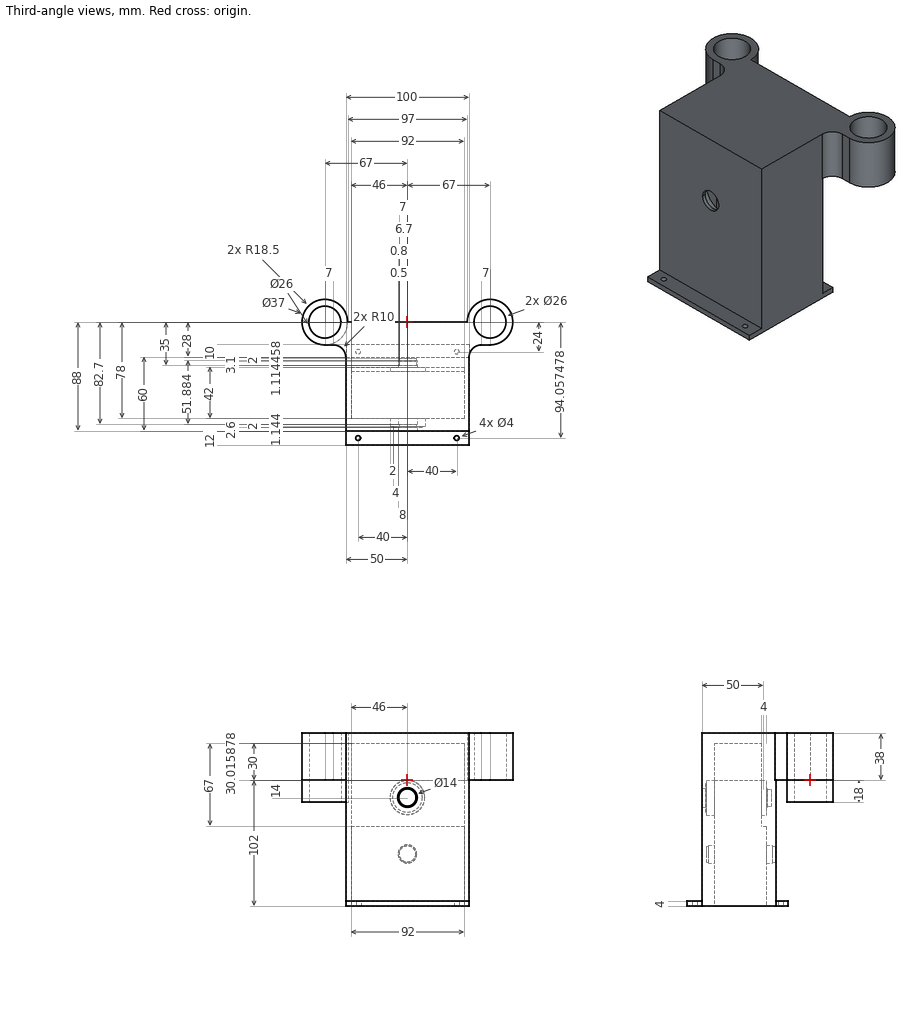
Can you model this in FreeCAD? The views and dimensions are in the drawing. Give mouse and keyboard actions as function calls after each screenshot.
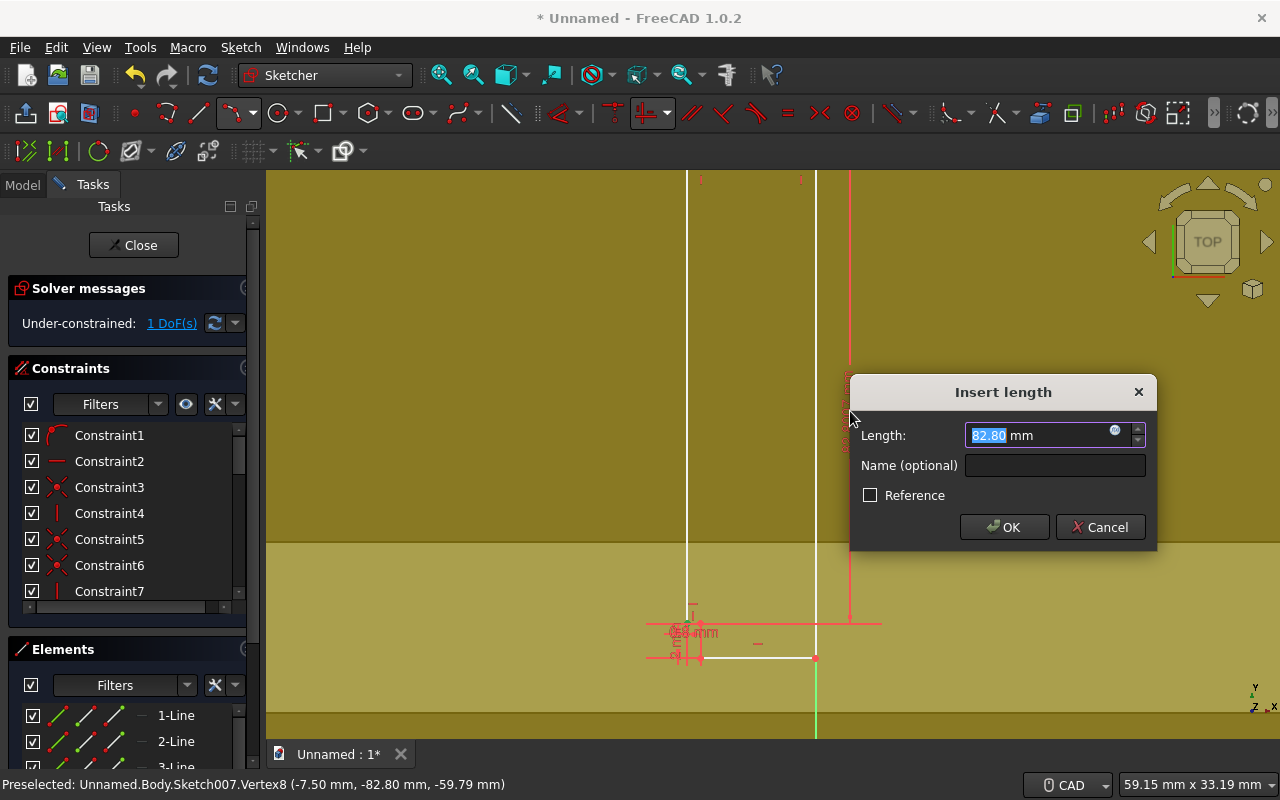
text(82.7)
key(Return)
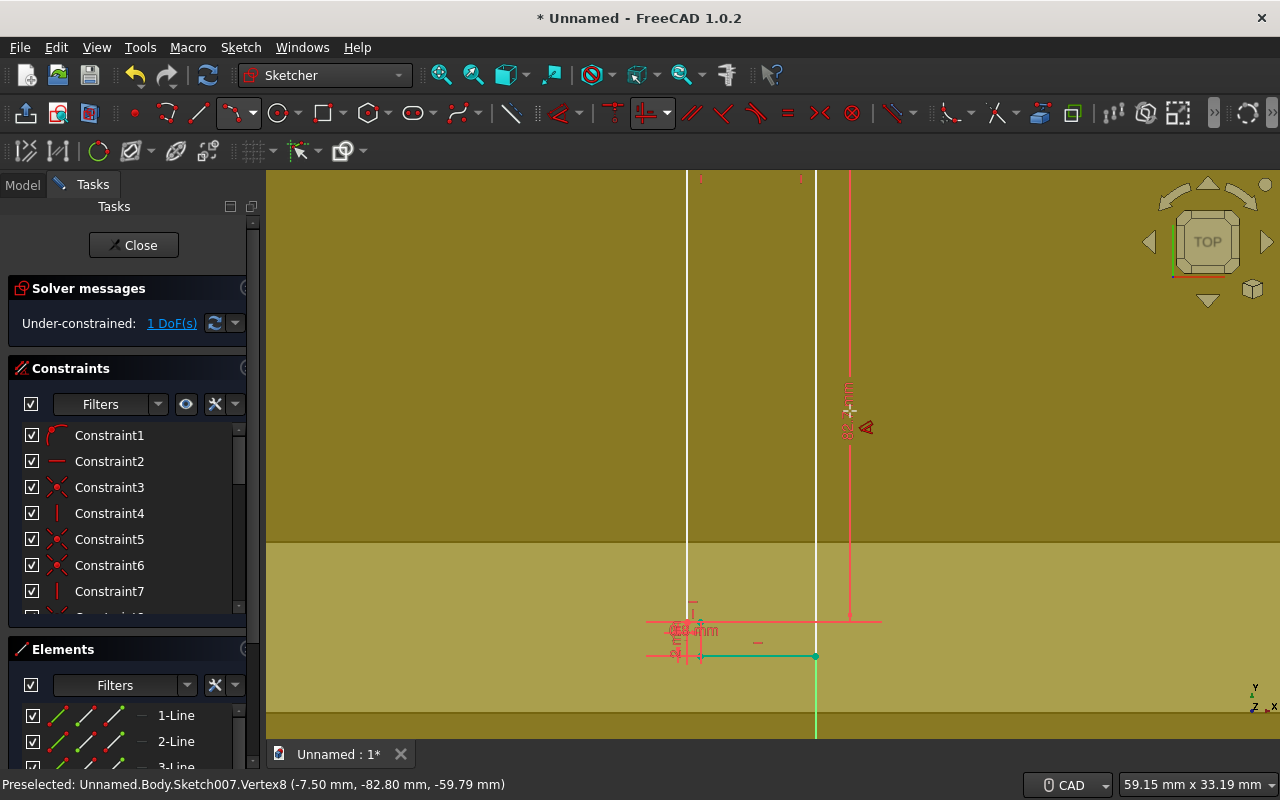
scroll(689, 626, down, 7)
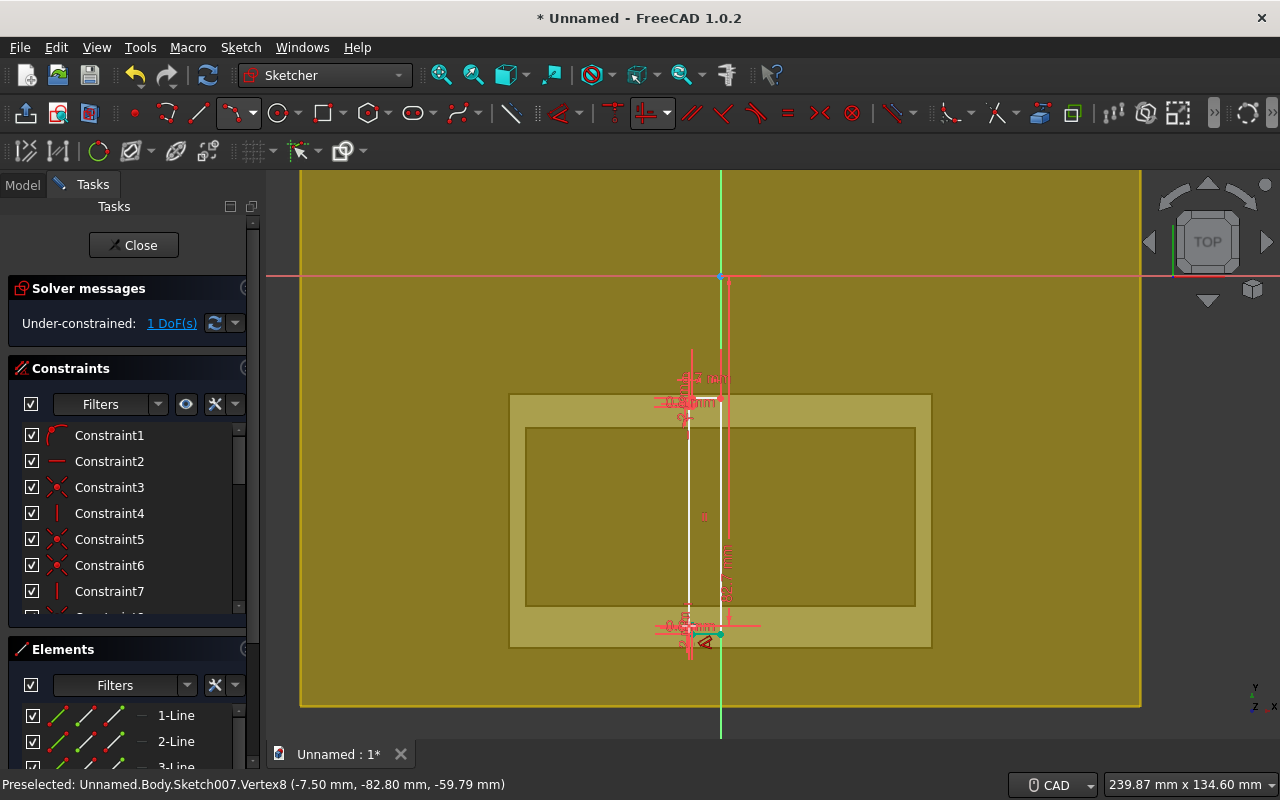
click(689, 560)
click(655, 516)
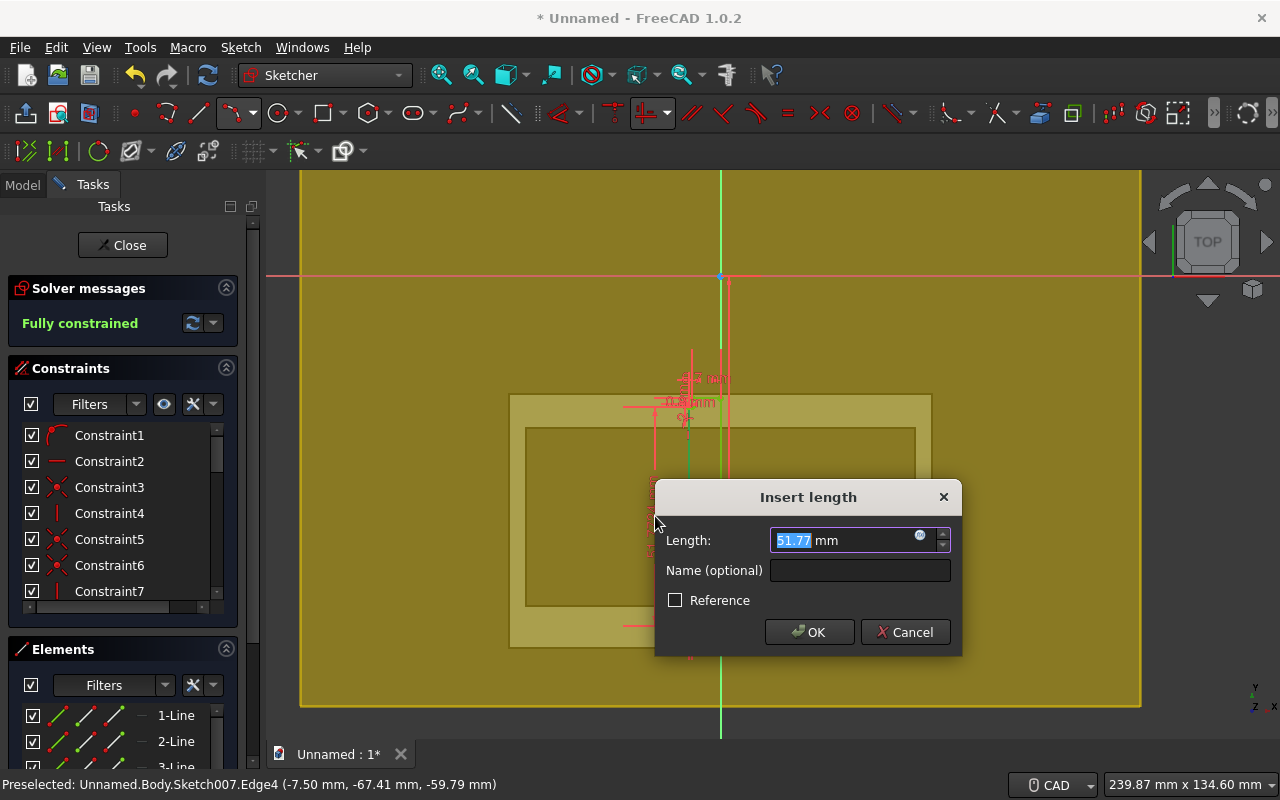
text(51.884)
key(Return)
key(Escape)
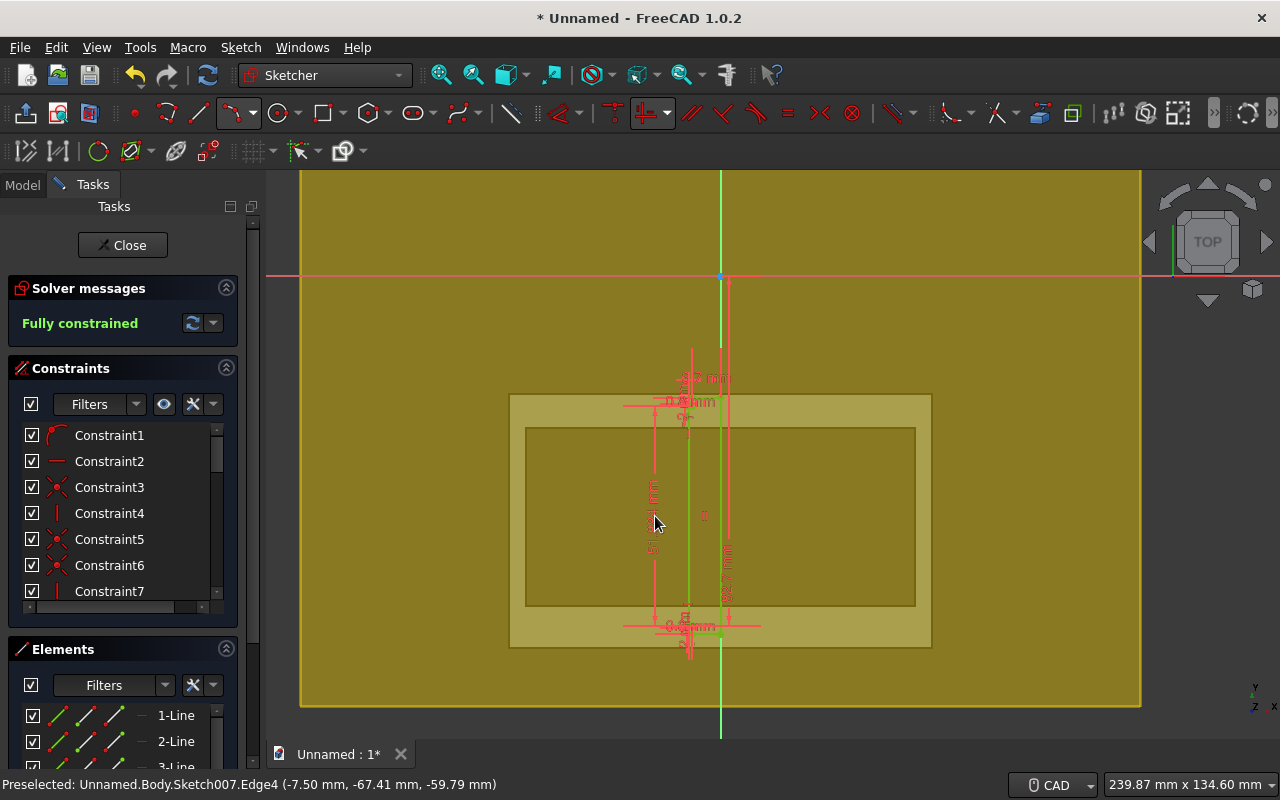
click(123, 245)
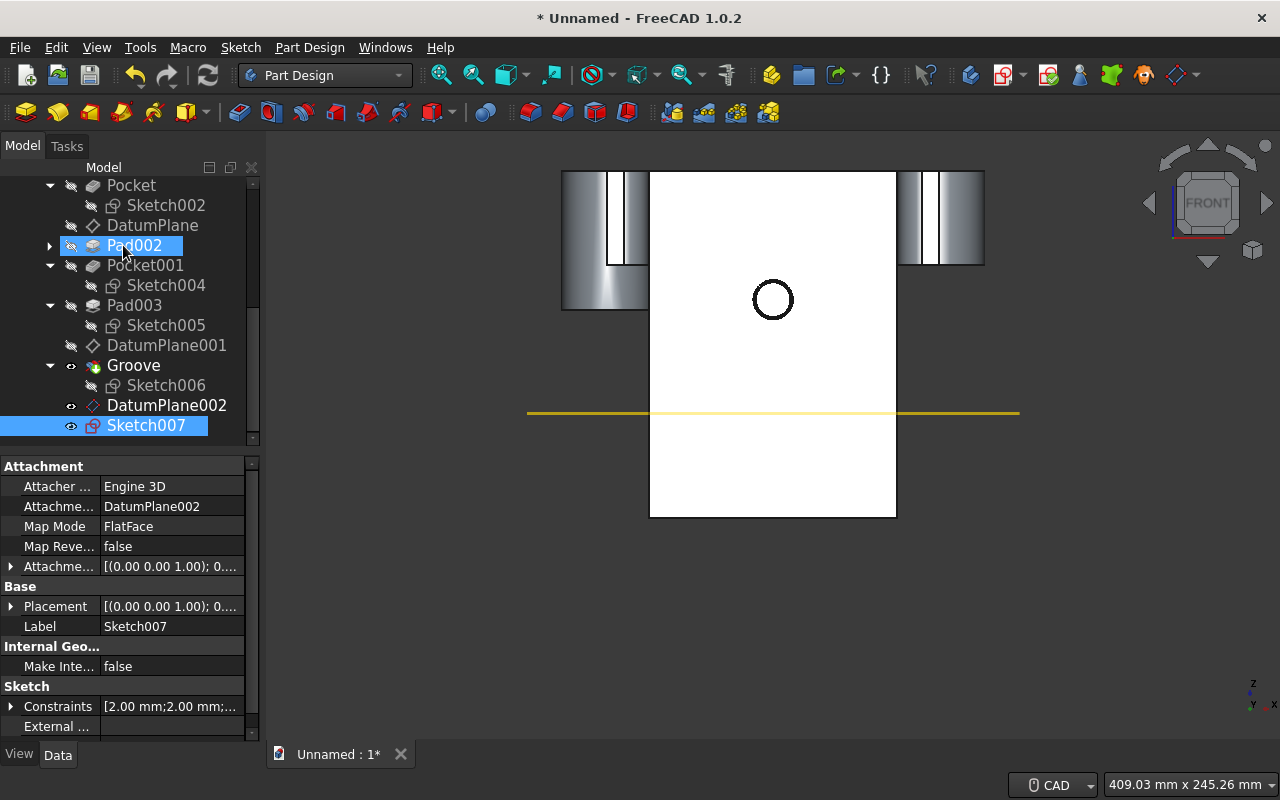
click(304, 112)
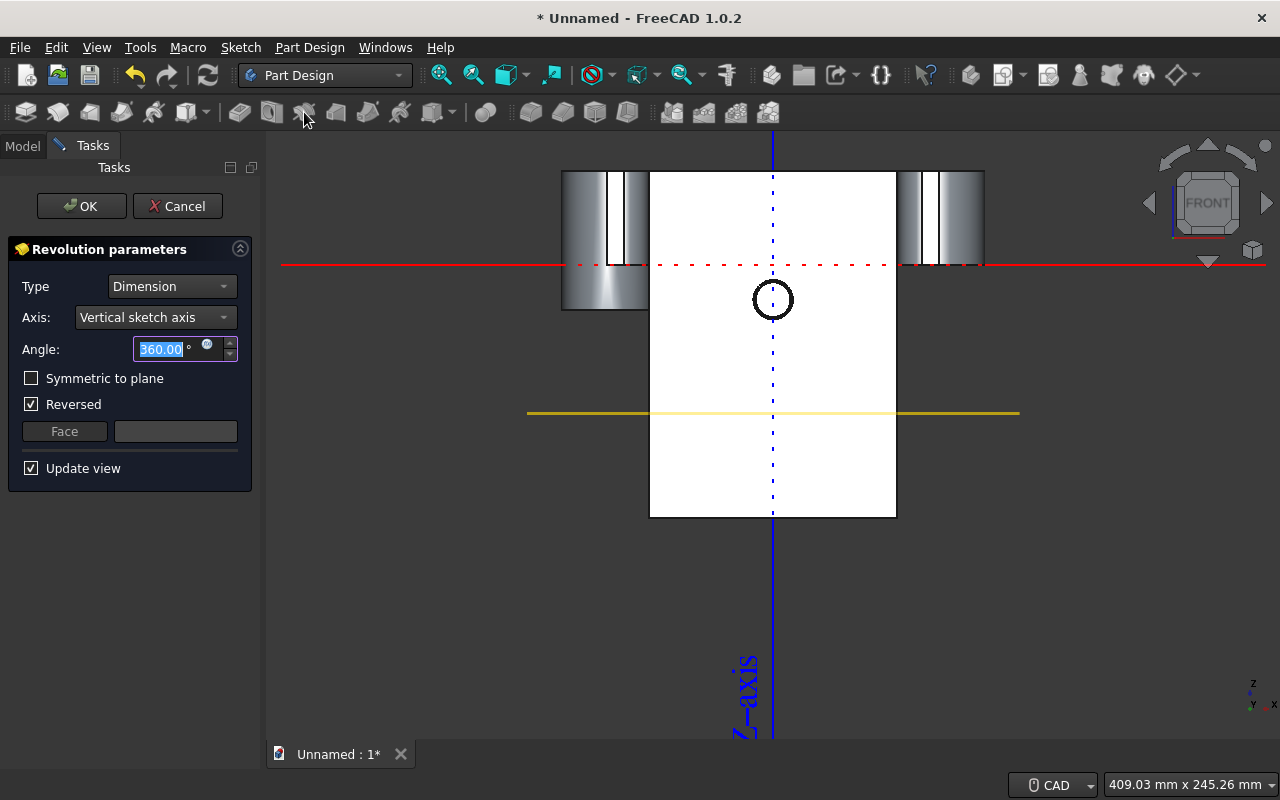
click(82, 206)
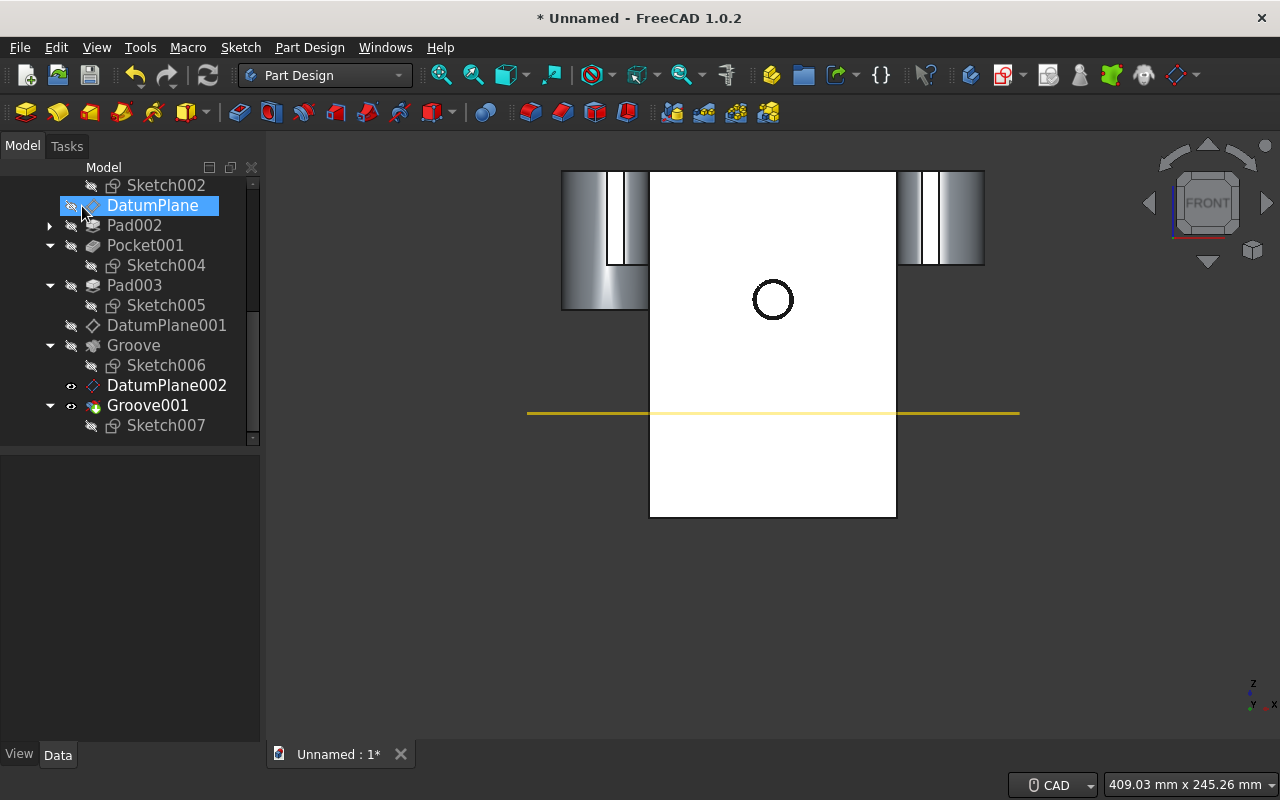
click(116, 386)
key(space)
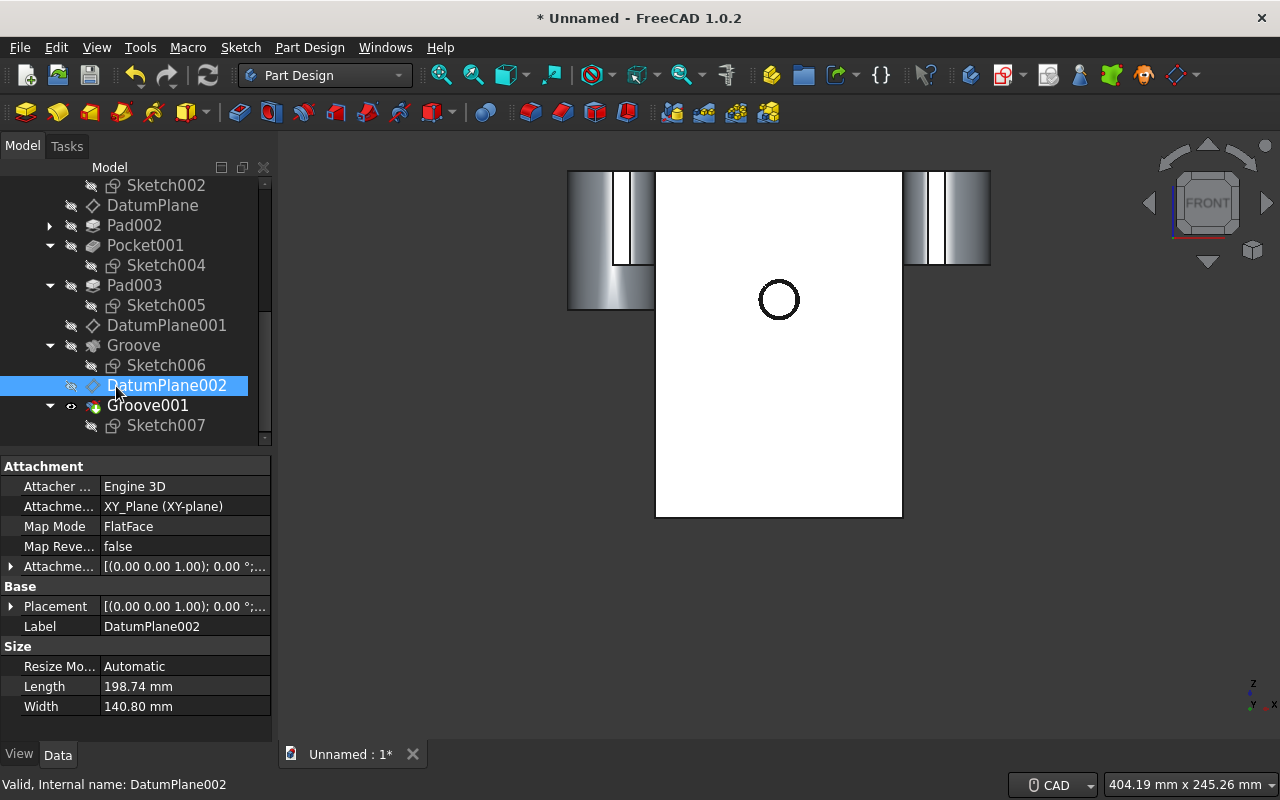
key(5)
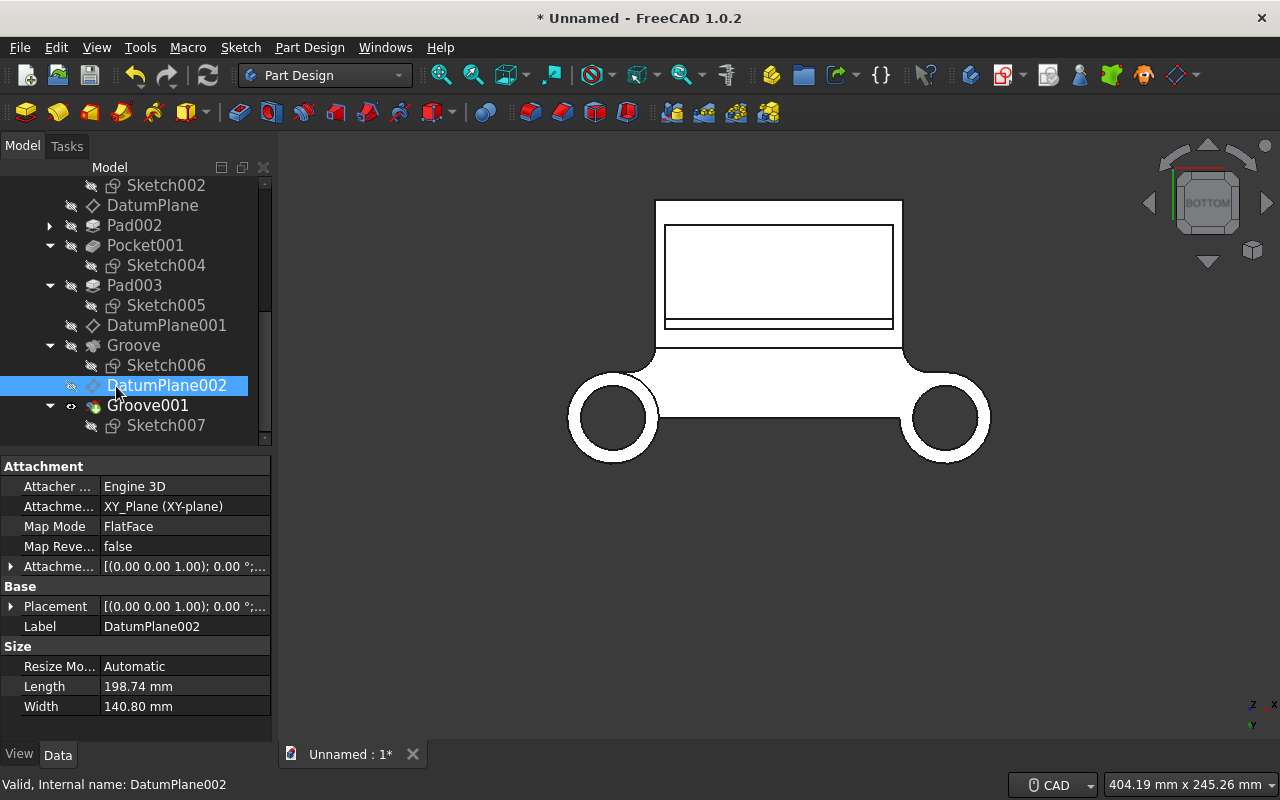
click(442, 76)